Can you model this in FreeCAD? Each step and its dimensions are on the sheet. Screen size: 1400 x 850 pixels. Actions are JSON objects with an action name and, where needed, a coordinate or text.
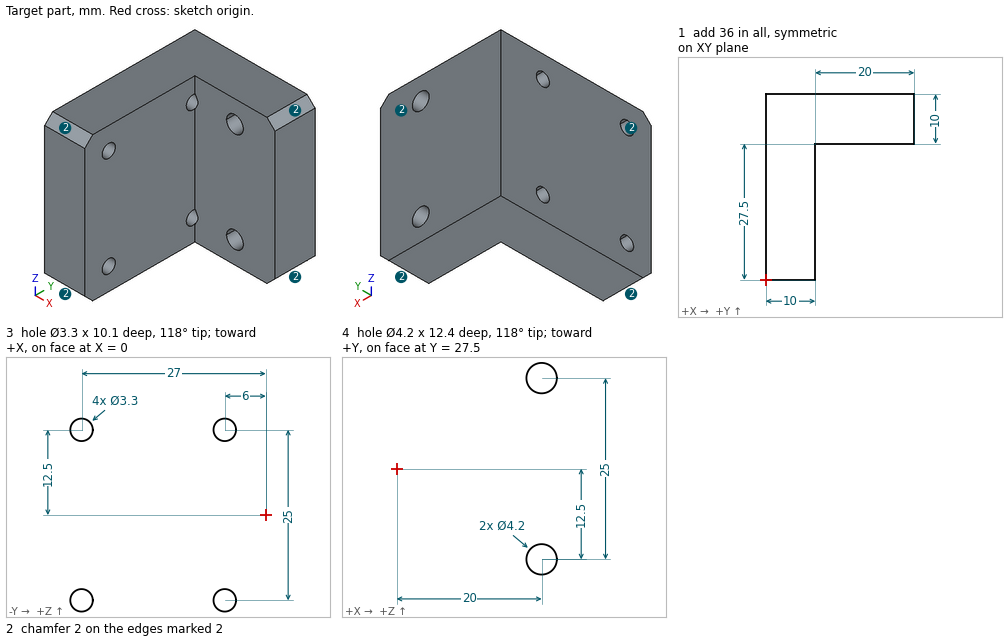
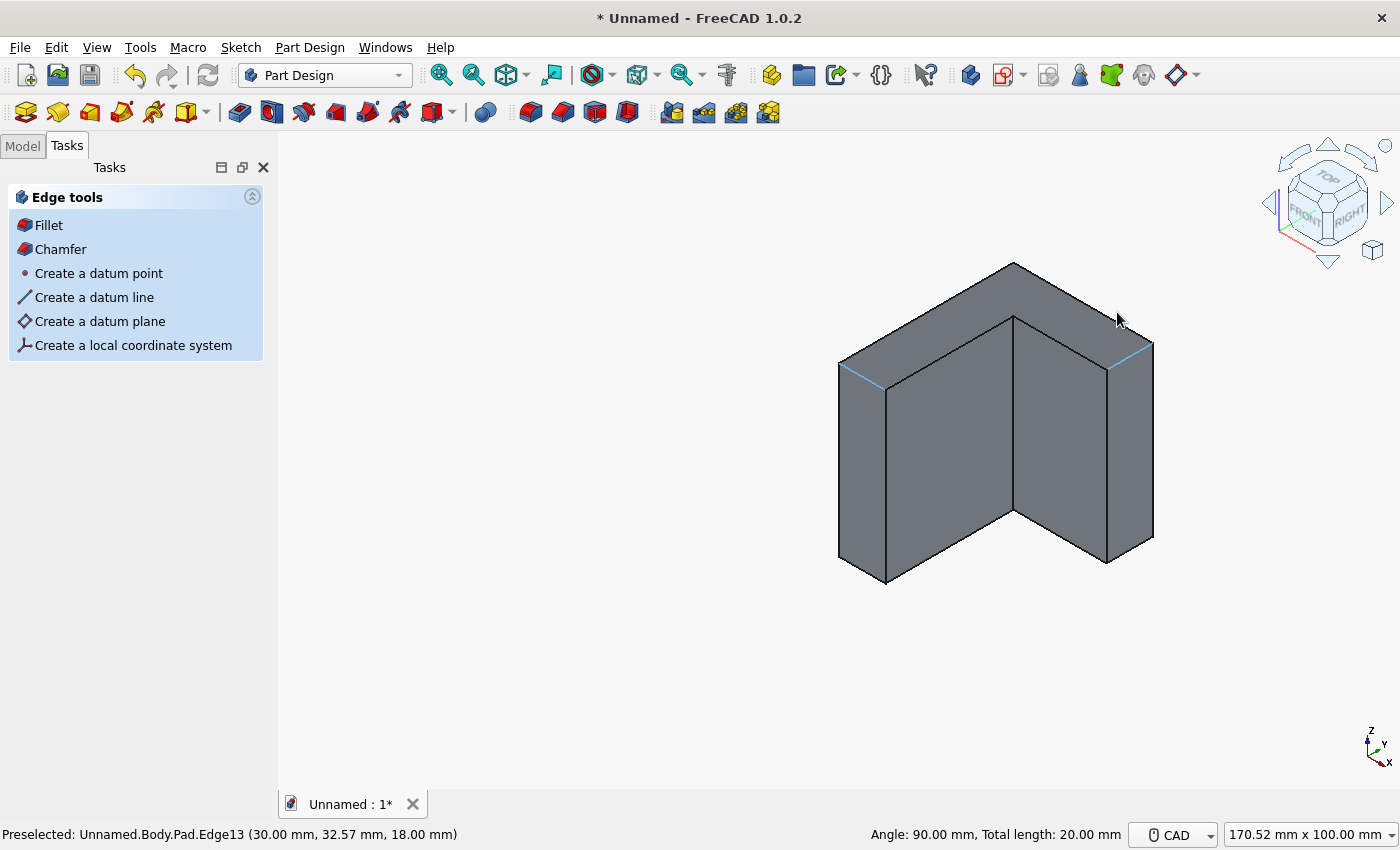
{"action": "key", "text": "2"}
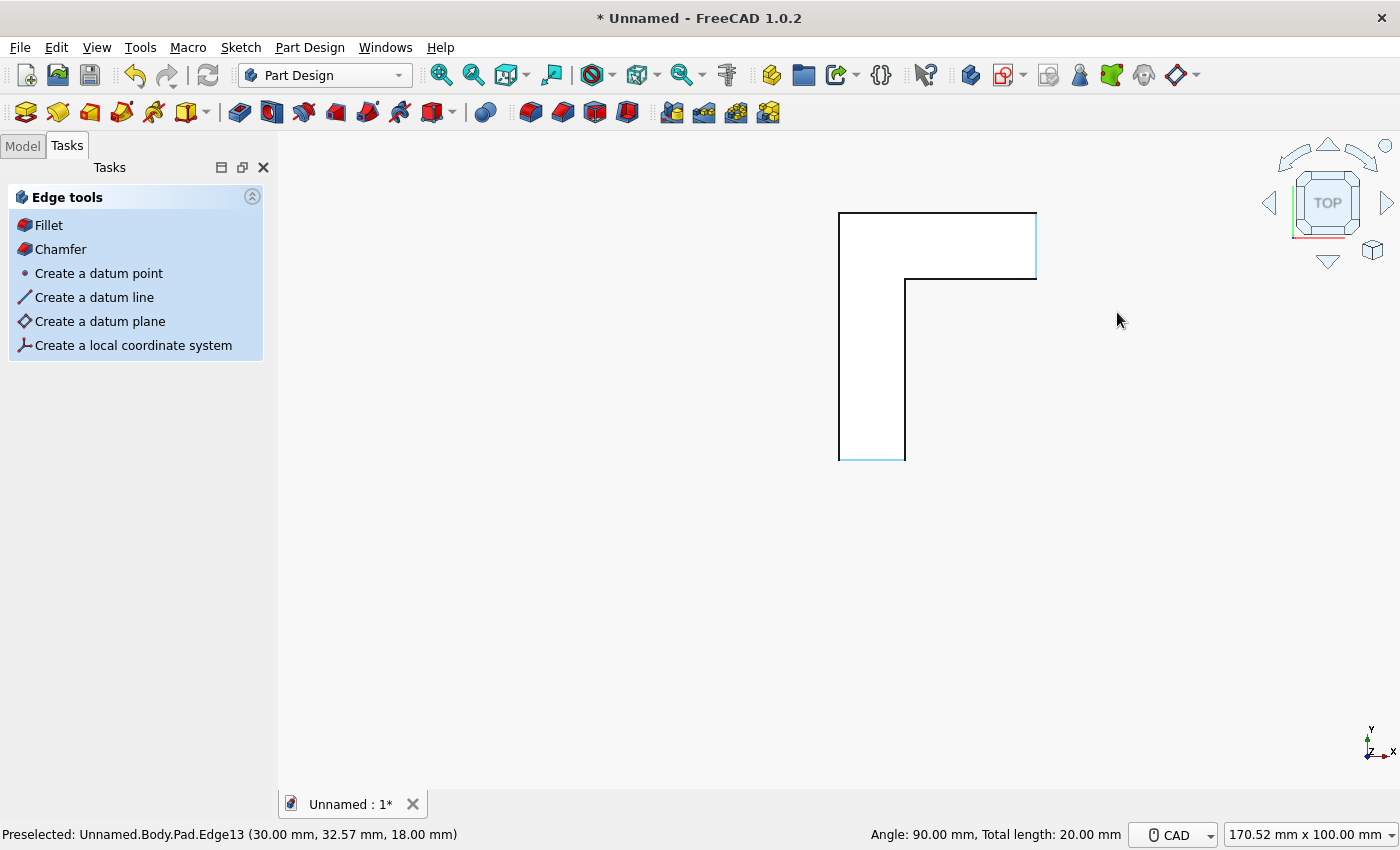
{"action": "key", "text": "v f"}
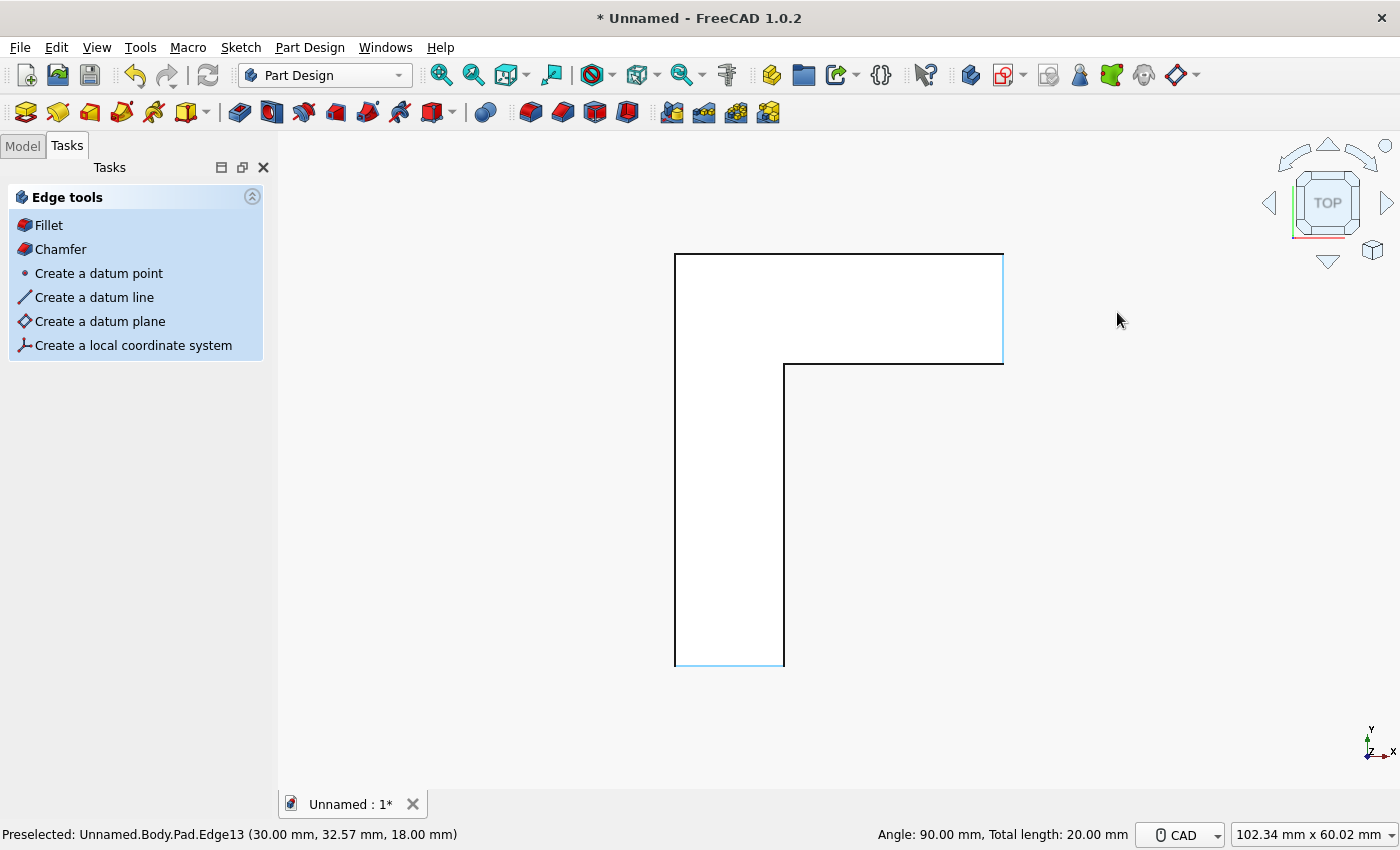
{"action": "key", "text": "1"}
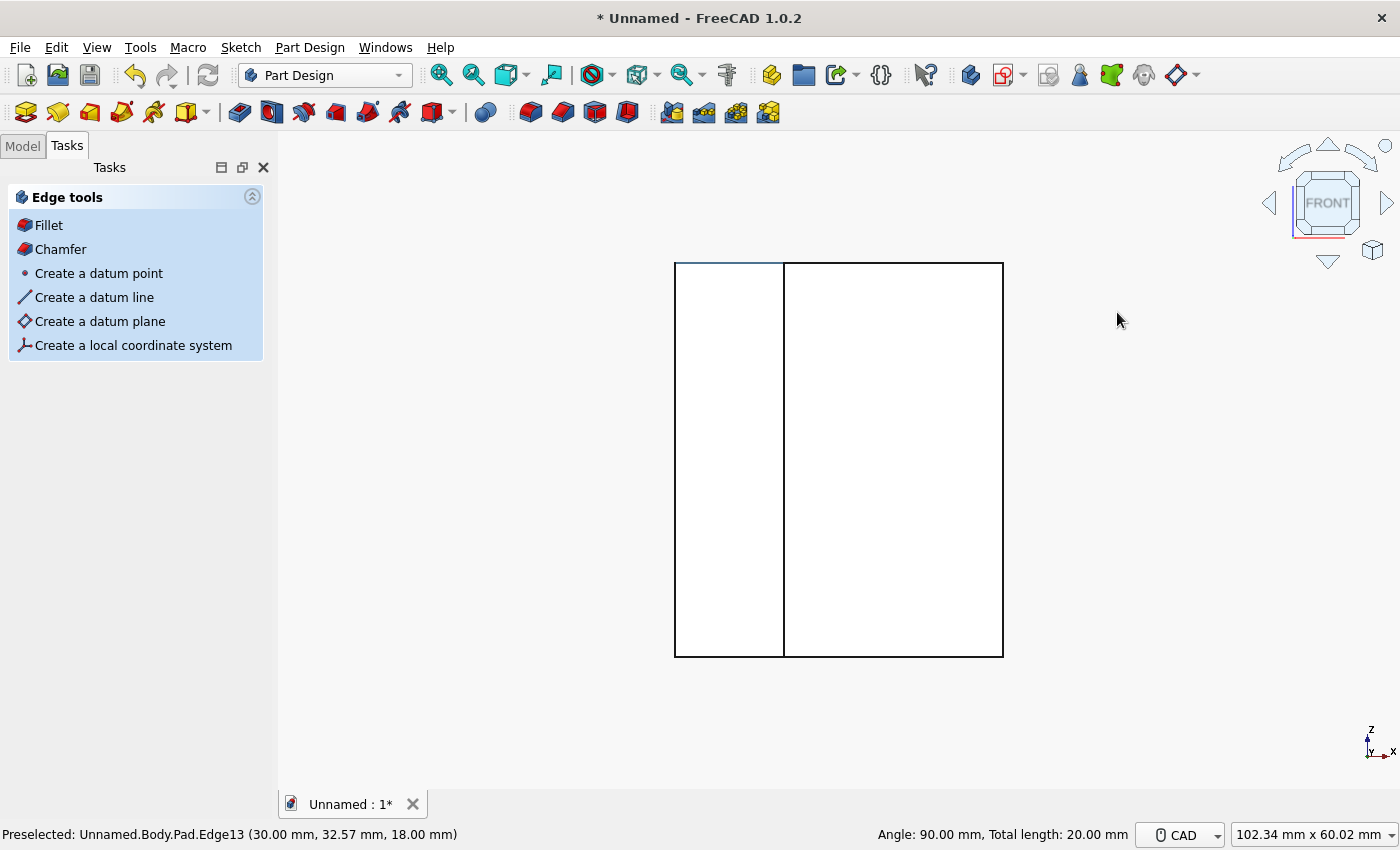
{"action": "left_click", "coordinate": [729, 656], "text": "ctrl"}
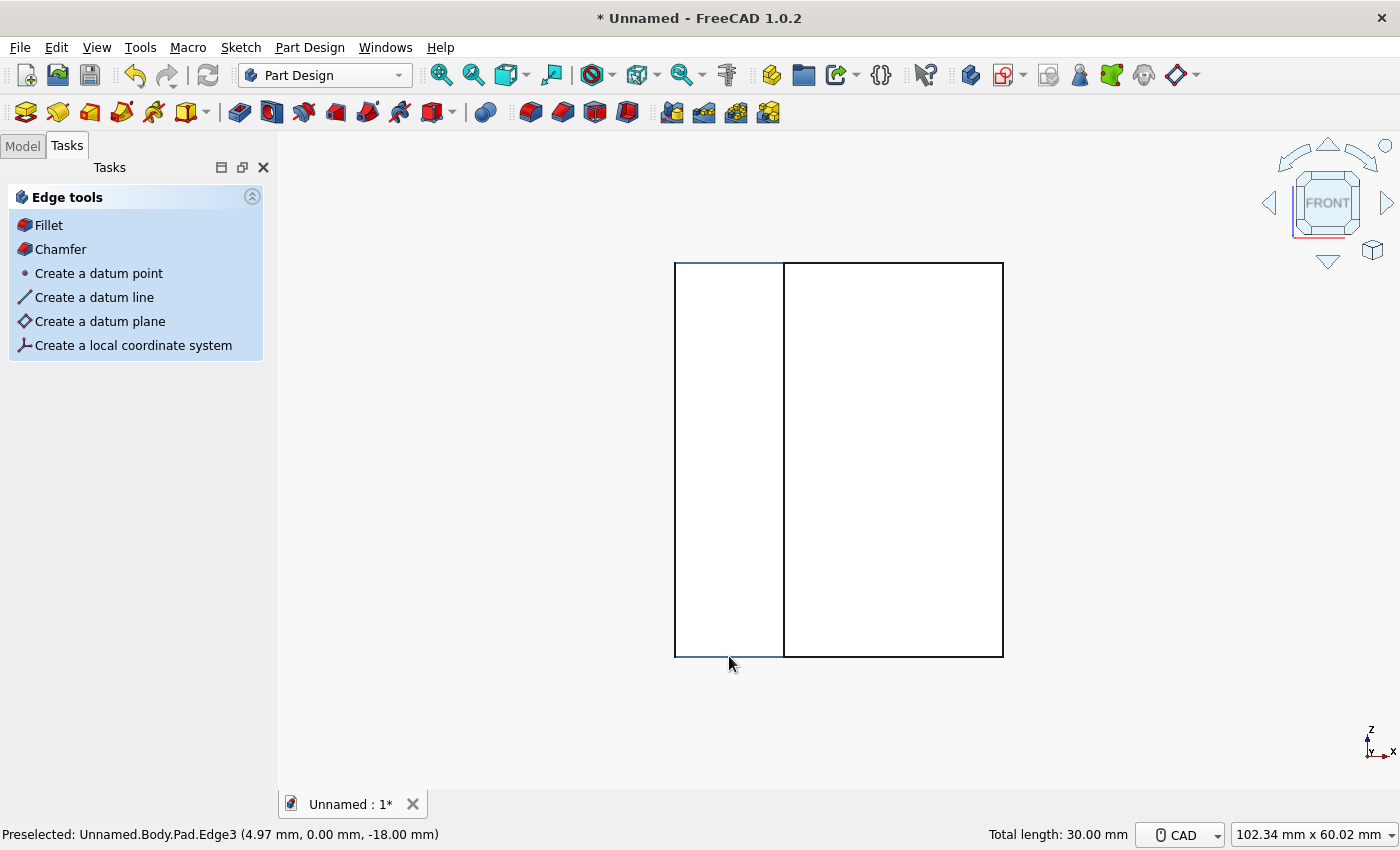
{"action": "key", "text": "3"}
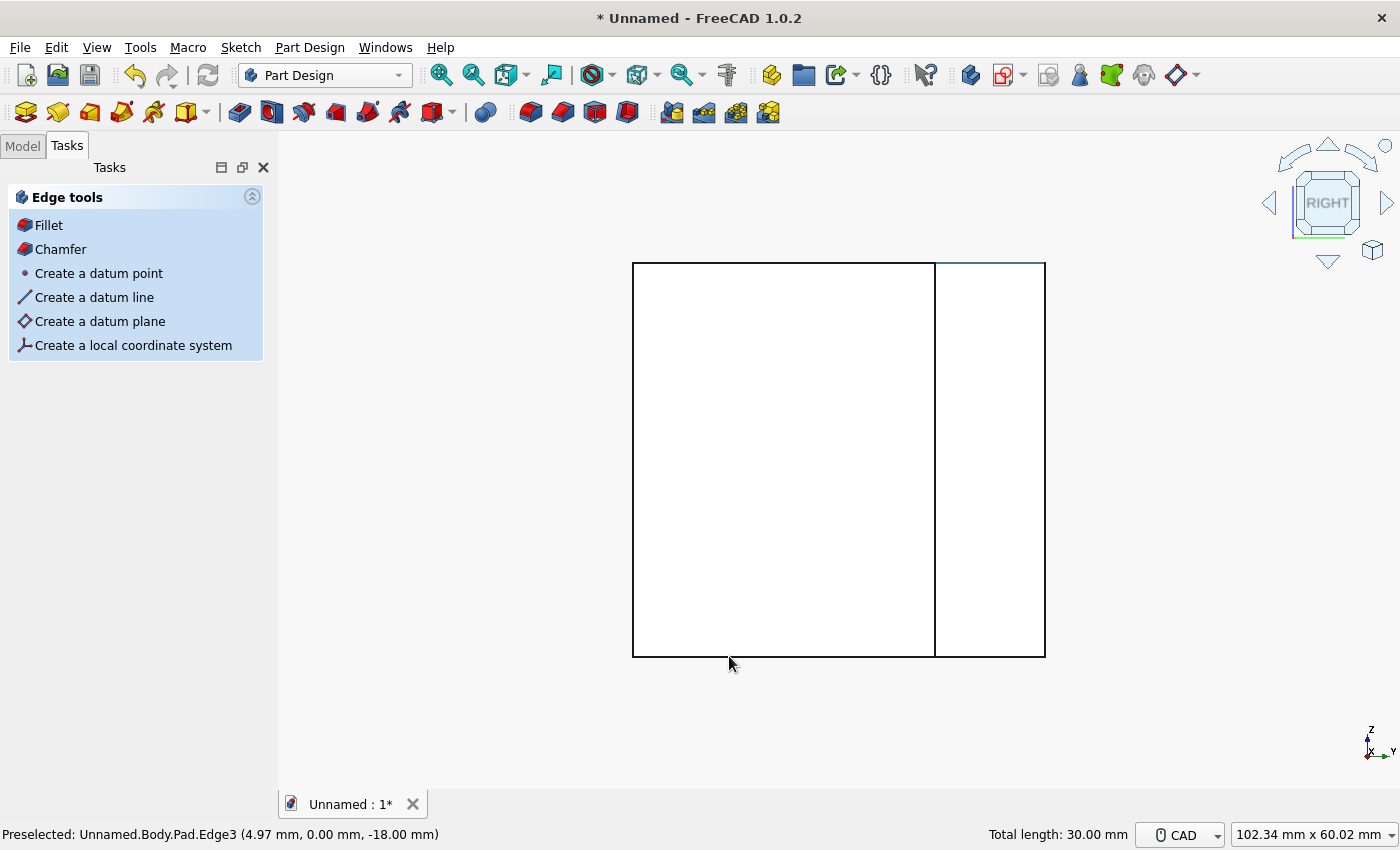
{"action": "left_click", "coordinate": [990, 656], "text": "ctrl"}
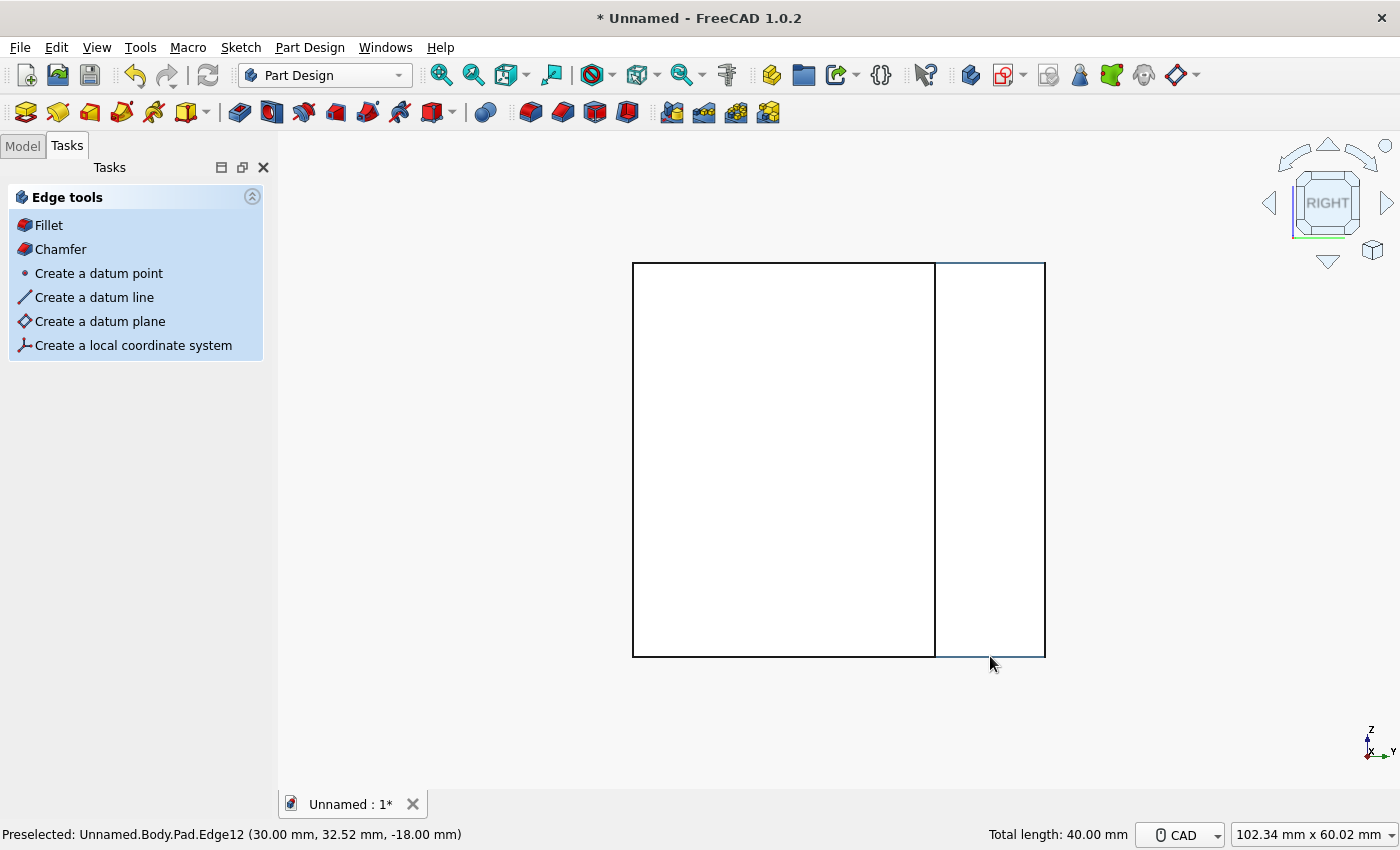
{"action": "left_click", "coordinate": [564, 112]}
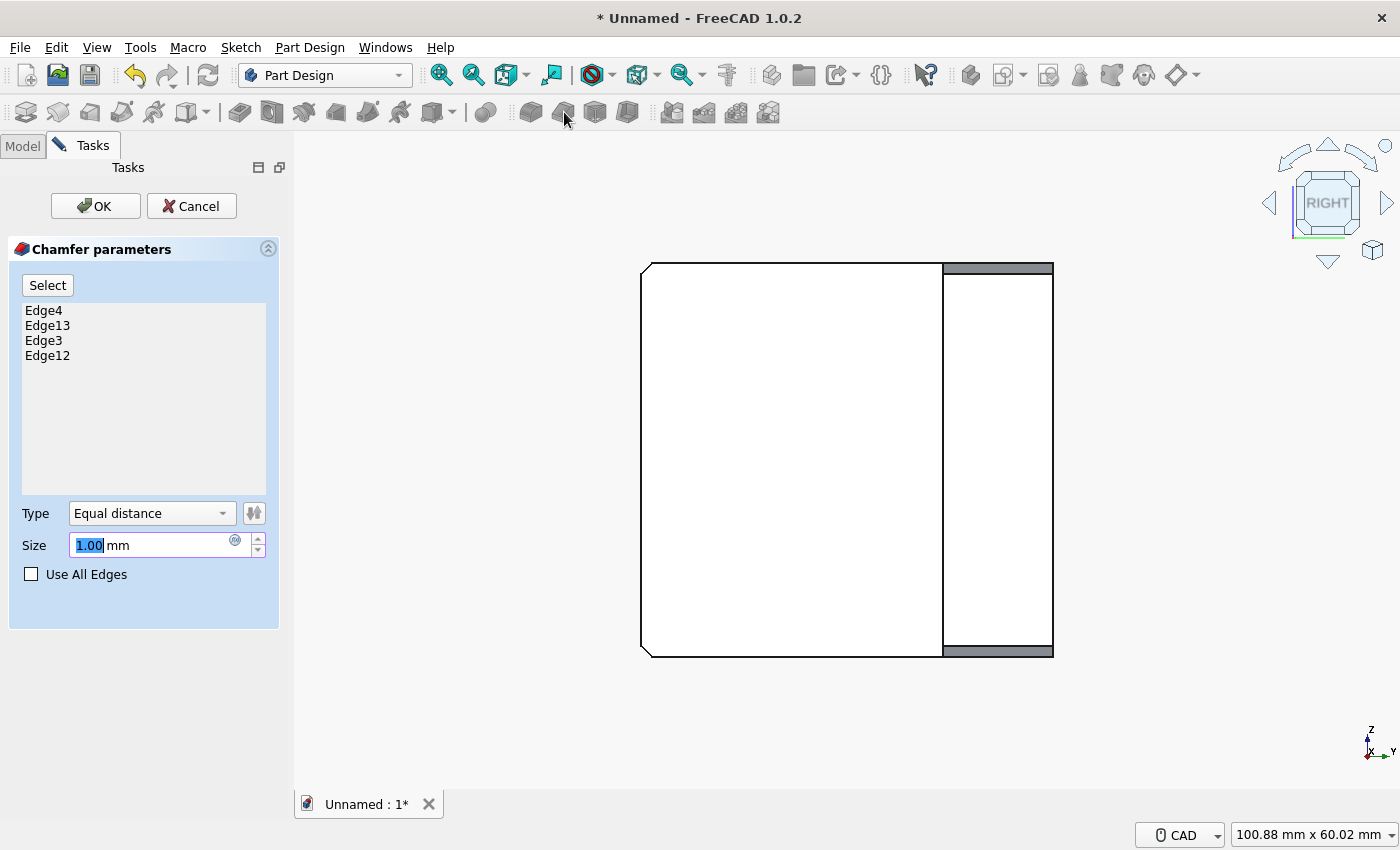
{"action": "type", "text": "2"}
{"action": "key", "text": "Tab"}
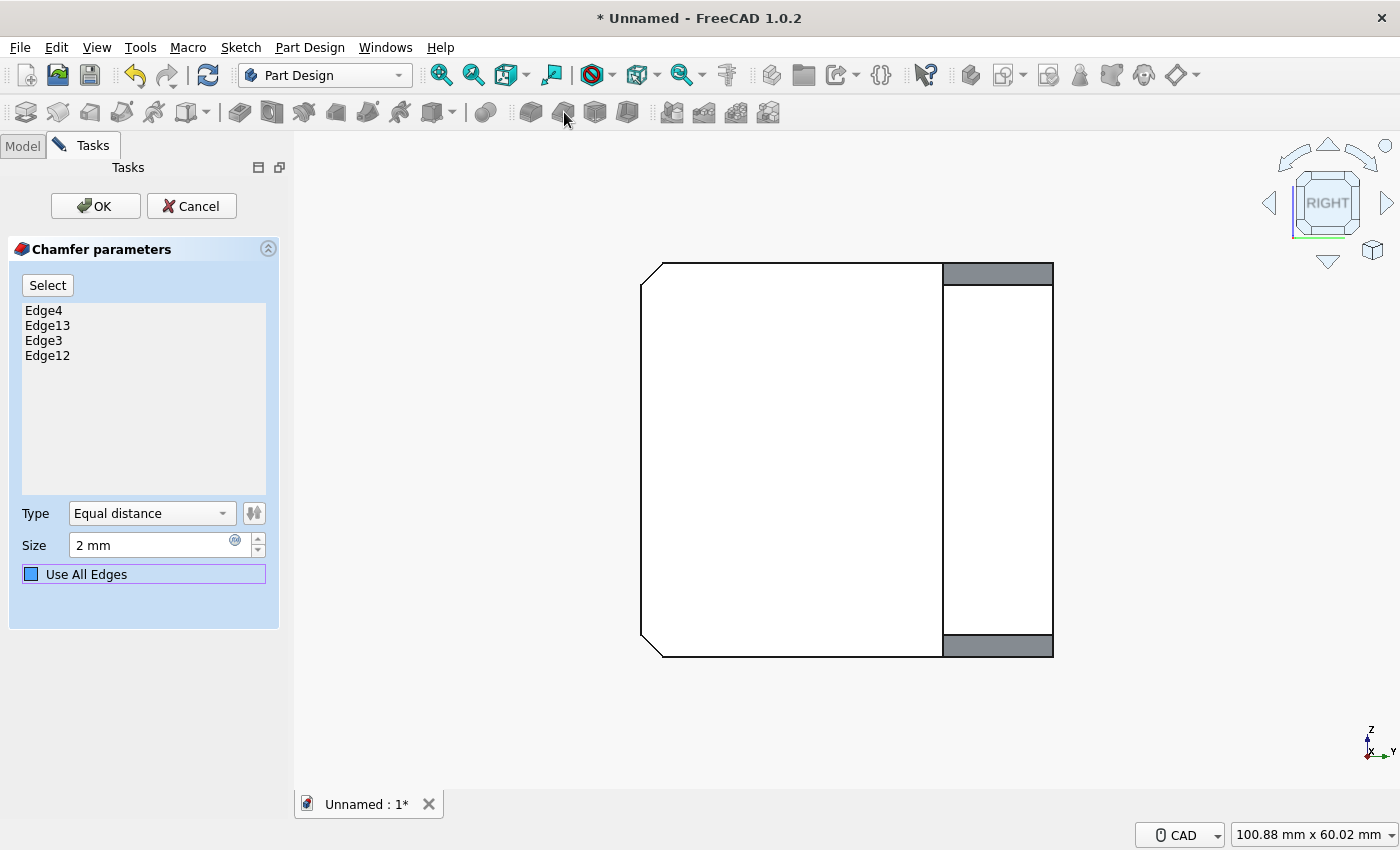
{"action": "left_click", "coordinate": [96, 206]}